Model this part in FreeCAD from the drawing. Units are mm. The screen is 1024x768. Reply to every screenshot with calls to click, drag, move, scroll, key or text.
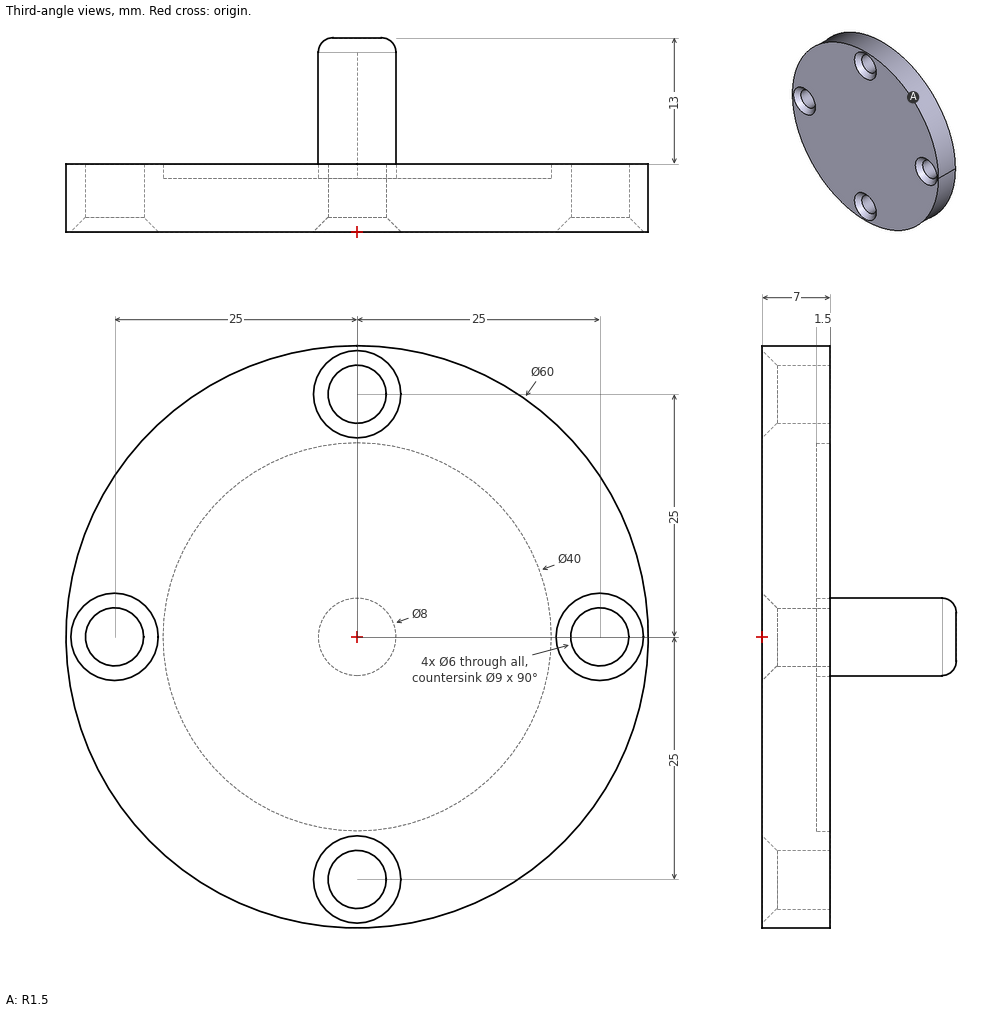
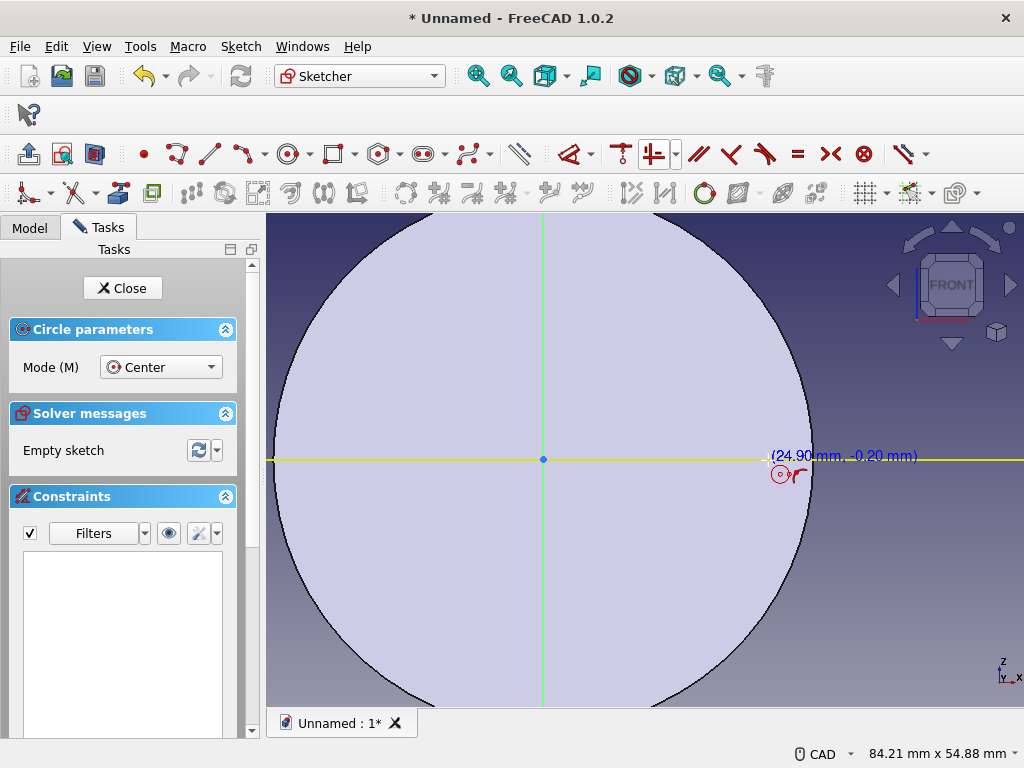
click(768, 460)
move(787, 440)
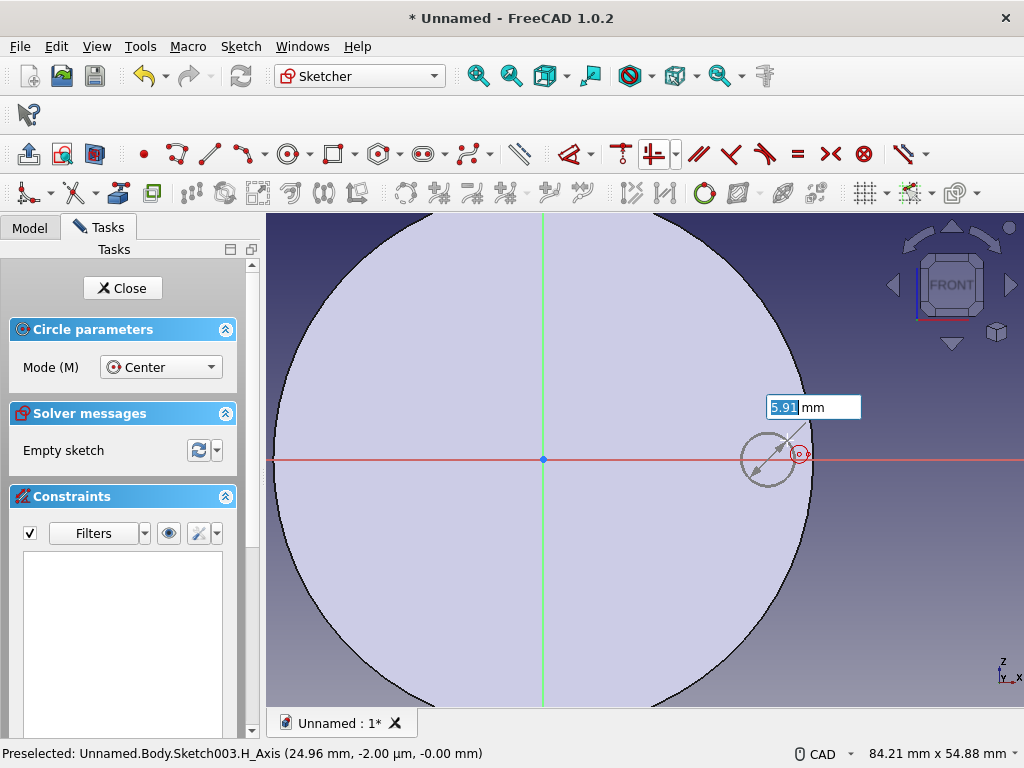
text(6)
key(Return)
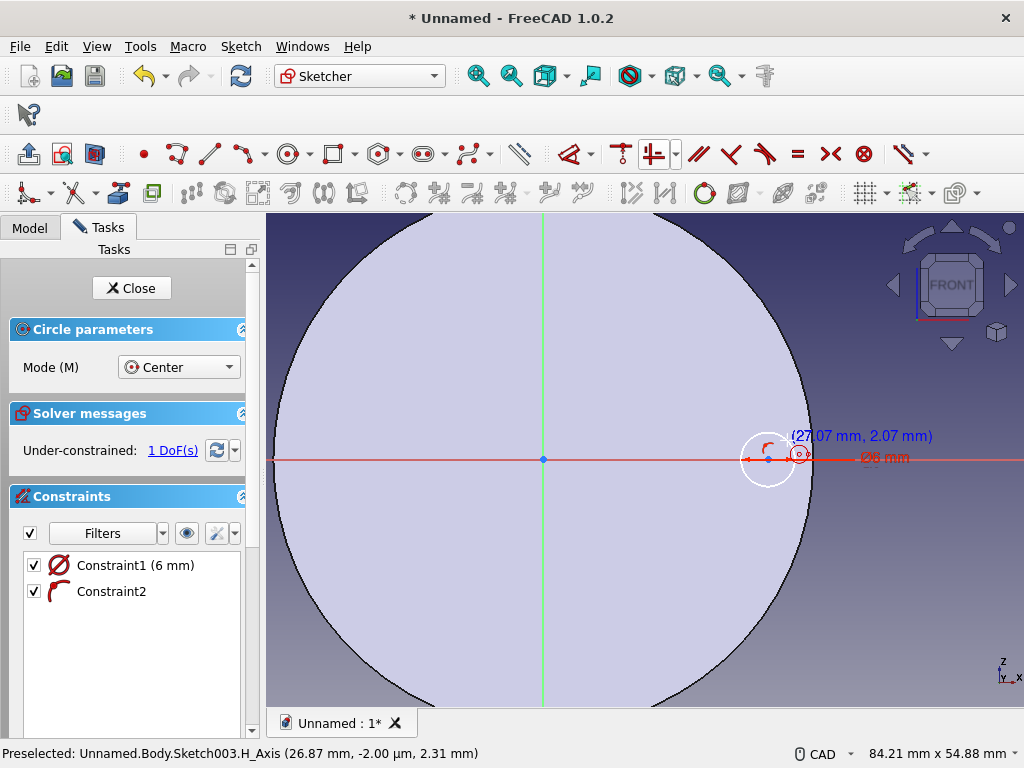
scroll(644, 461, down, 2)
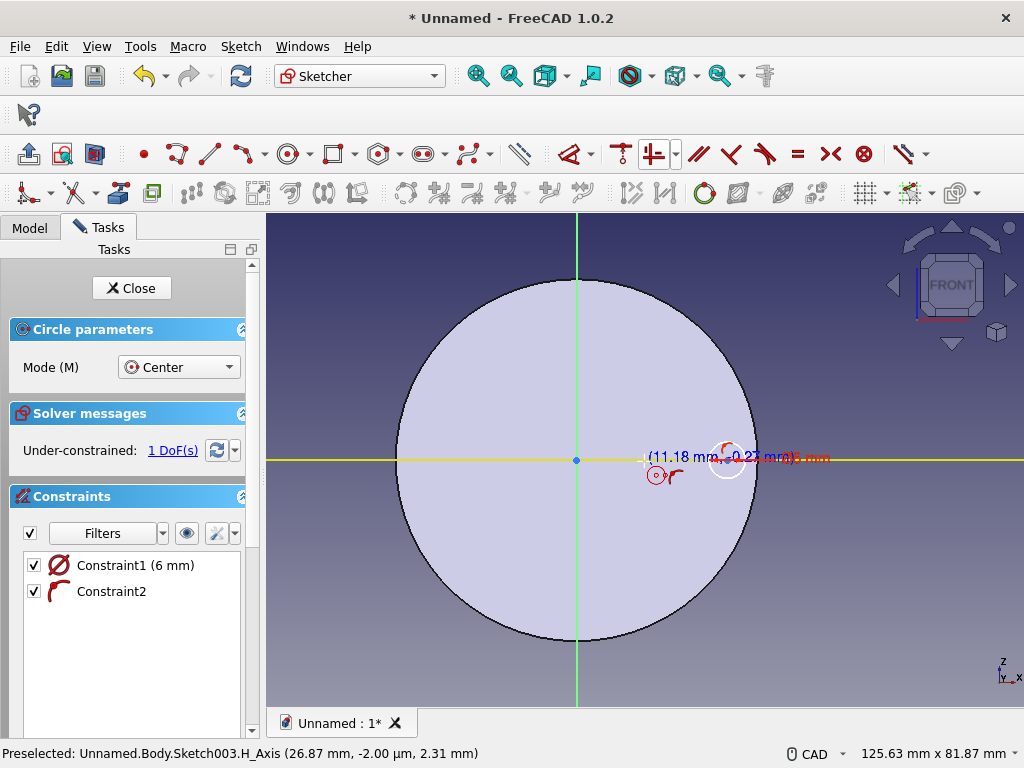
scroll(577, 611, up, 2)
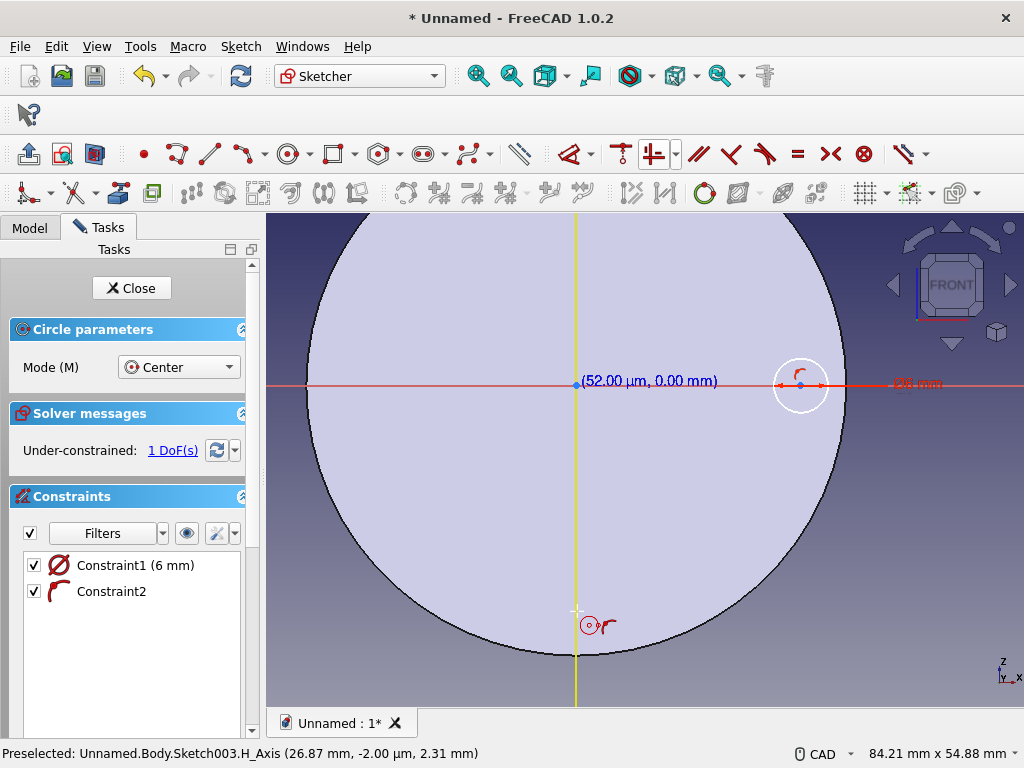
click(576, 611)
move(595, 592)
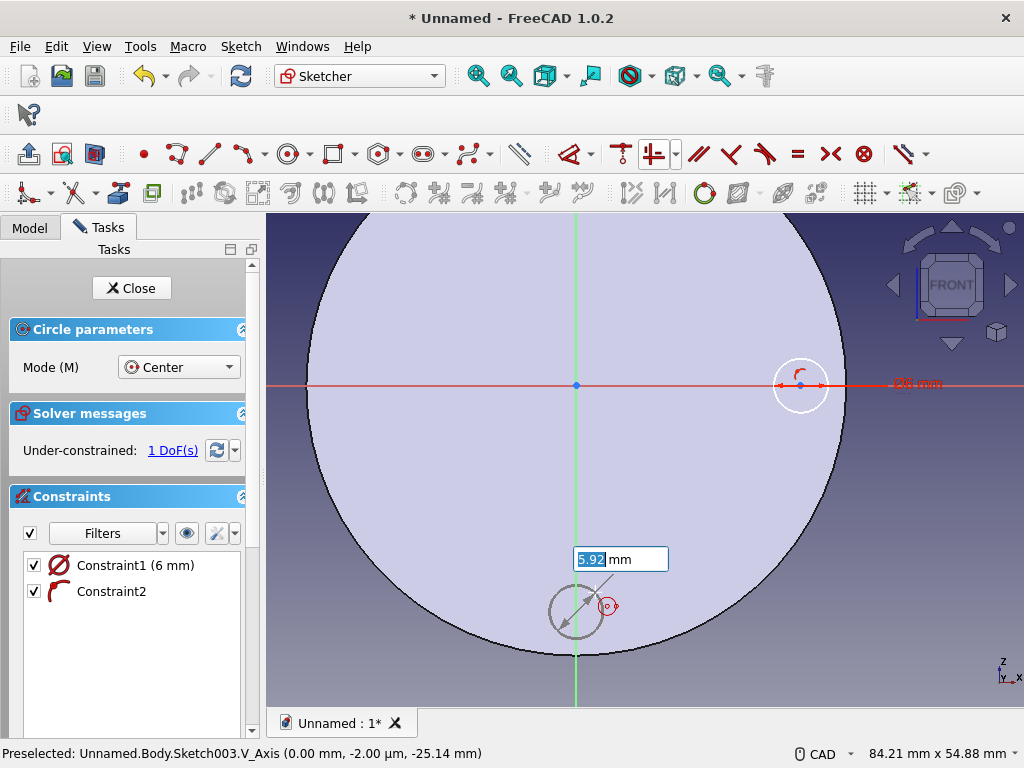
text(6)
key(Return)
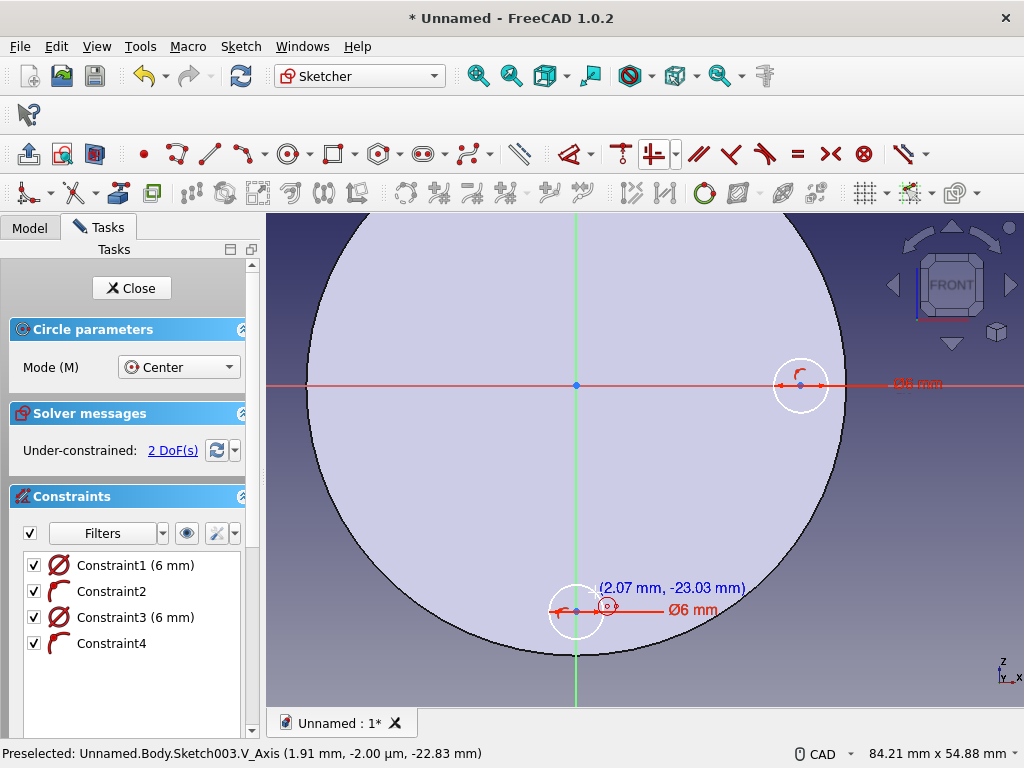
click(351, 386)
move(370, 367)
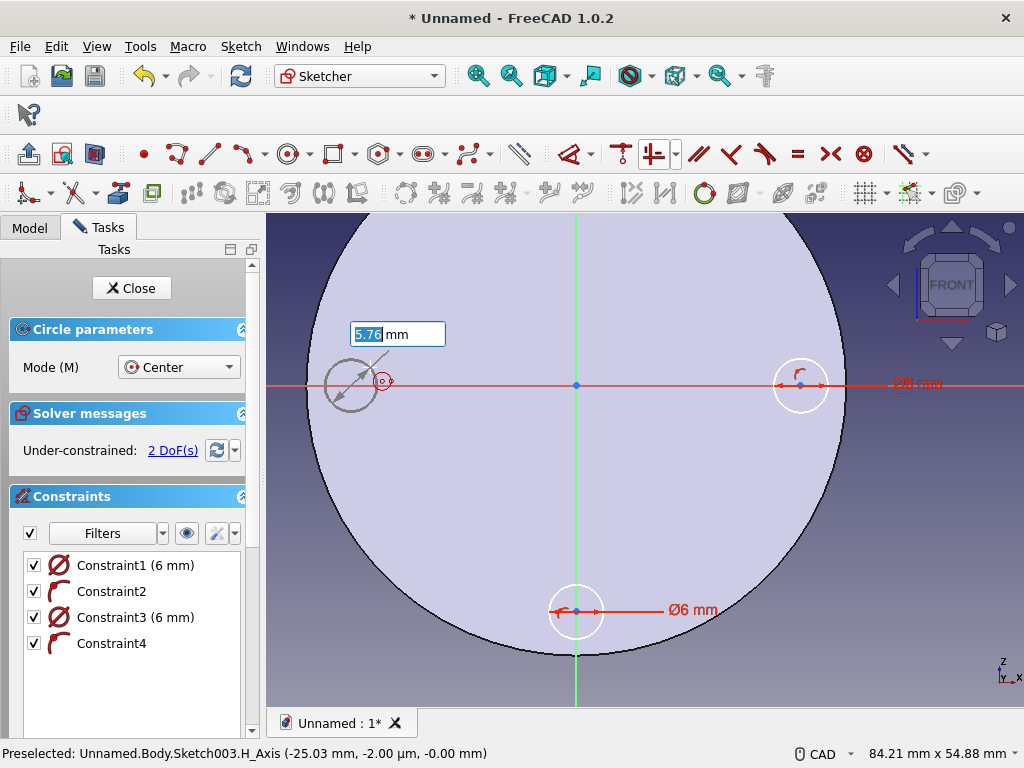
text(6)
key(Return)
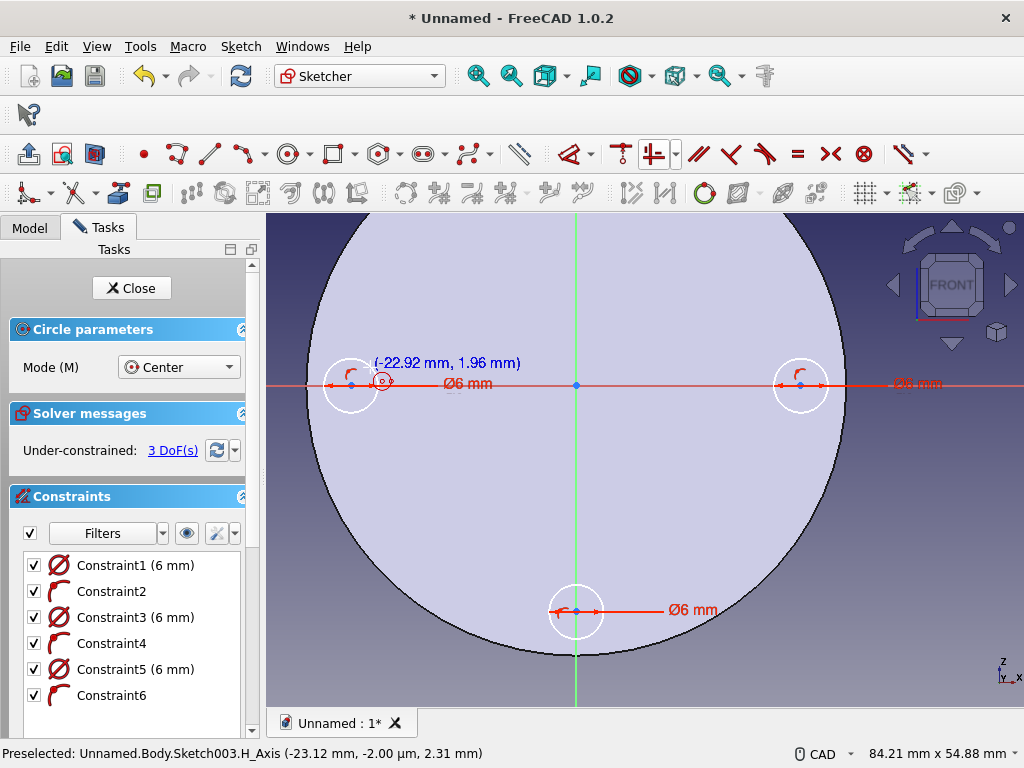
scroll(577, 611, down, 2)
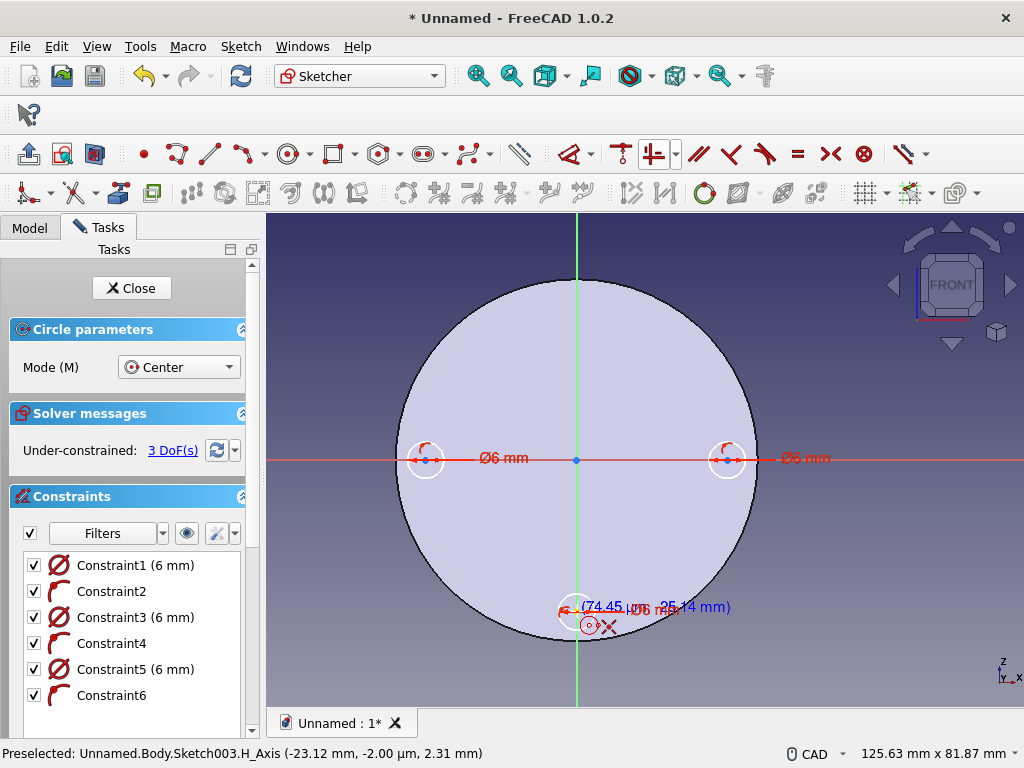
scroll(577, 309, up, 2)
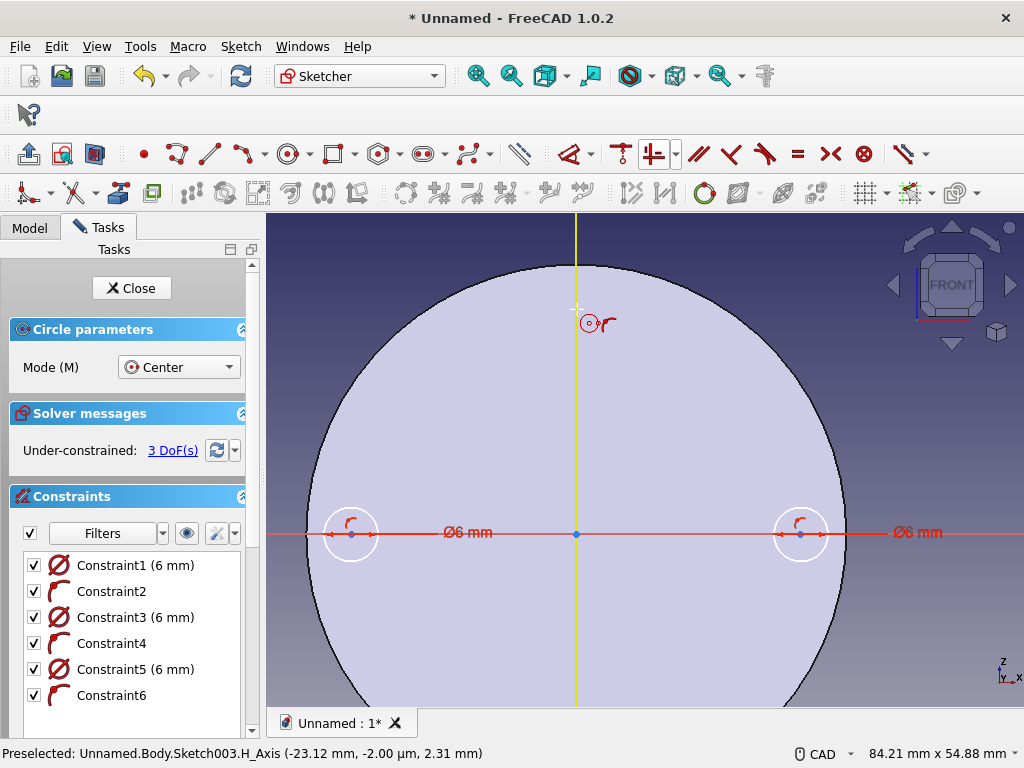
click(576, 309)
move(595, 290)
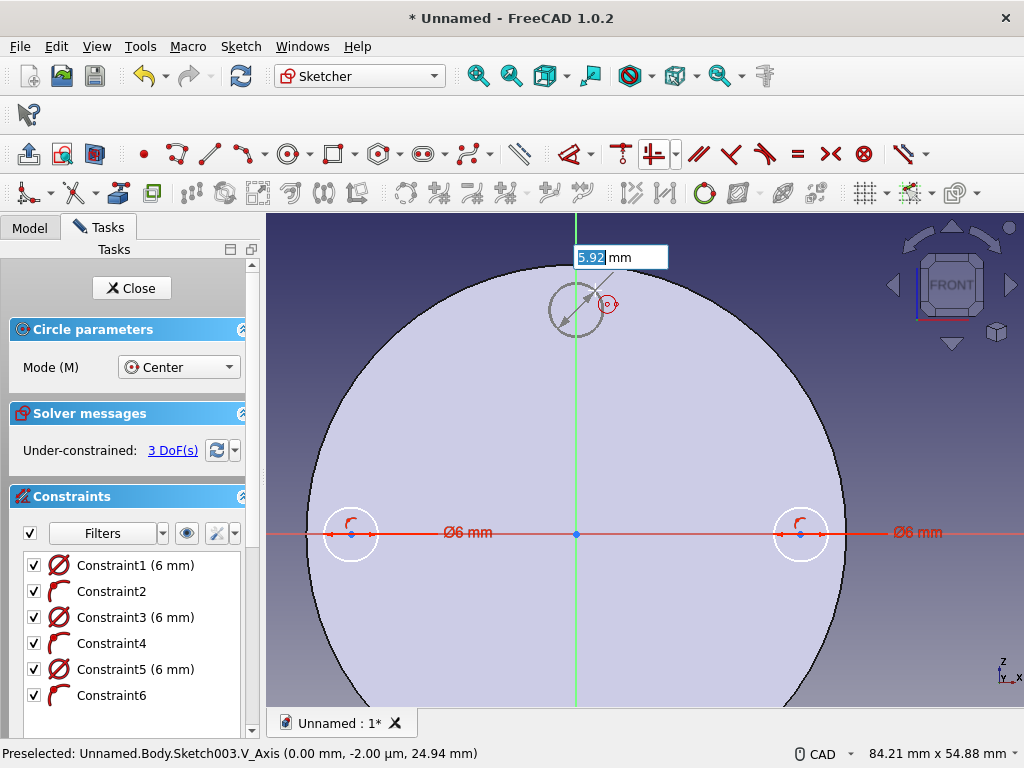
text(6)
key(Return)
key(Escape)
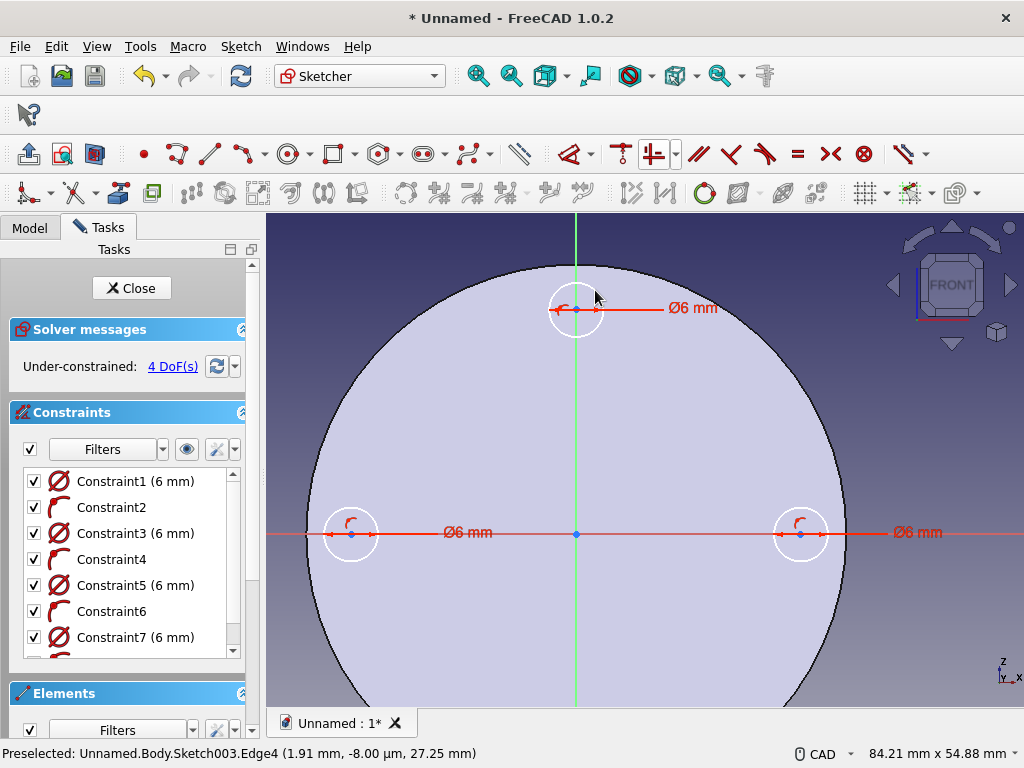
click(568, 154)